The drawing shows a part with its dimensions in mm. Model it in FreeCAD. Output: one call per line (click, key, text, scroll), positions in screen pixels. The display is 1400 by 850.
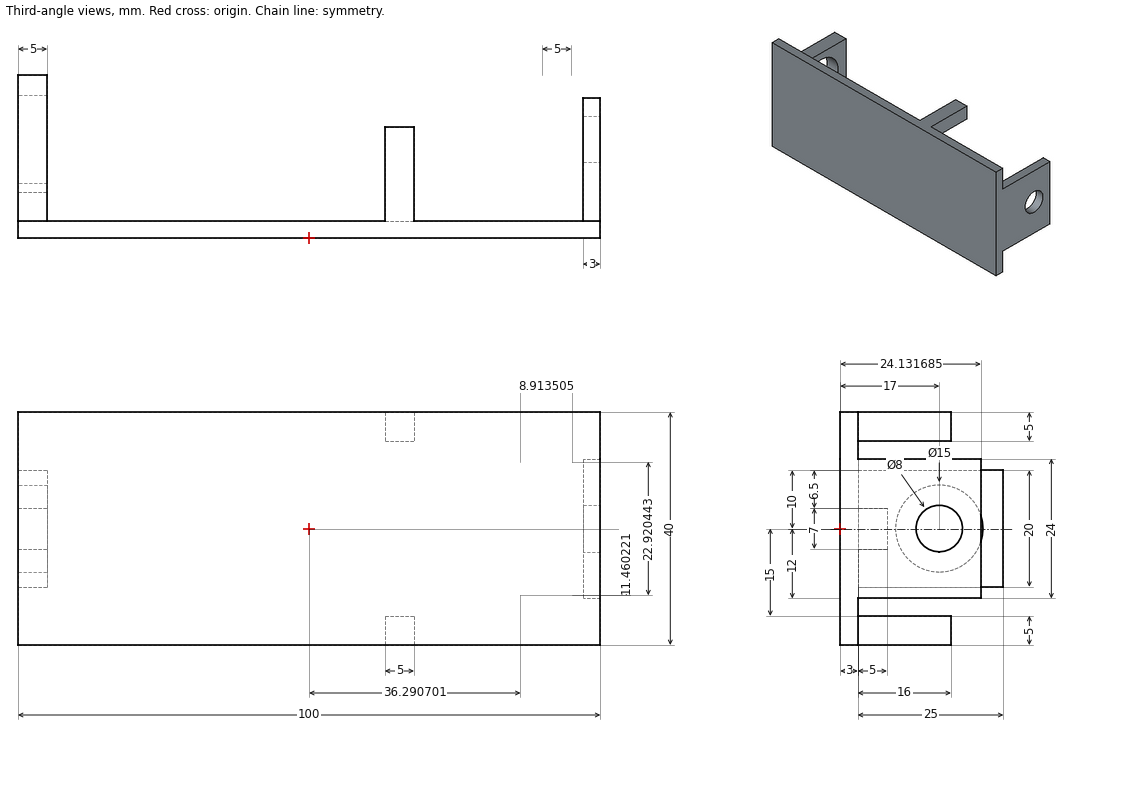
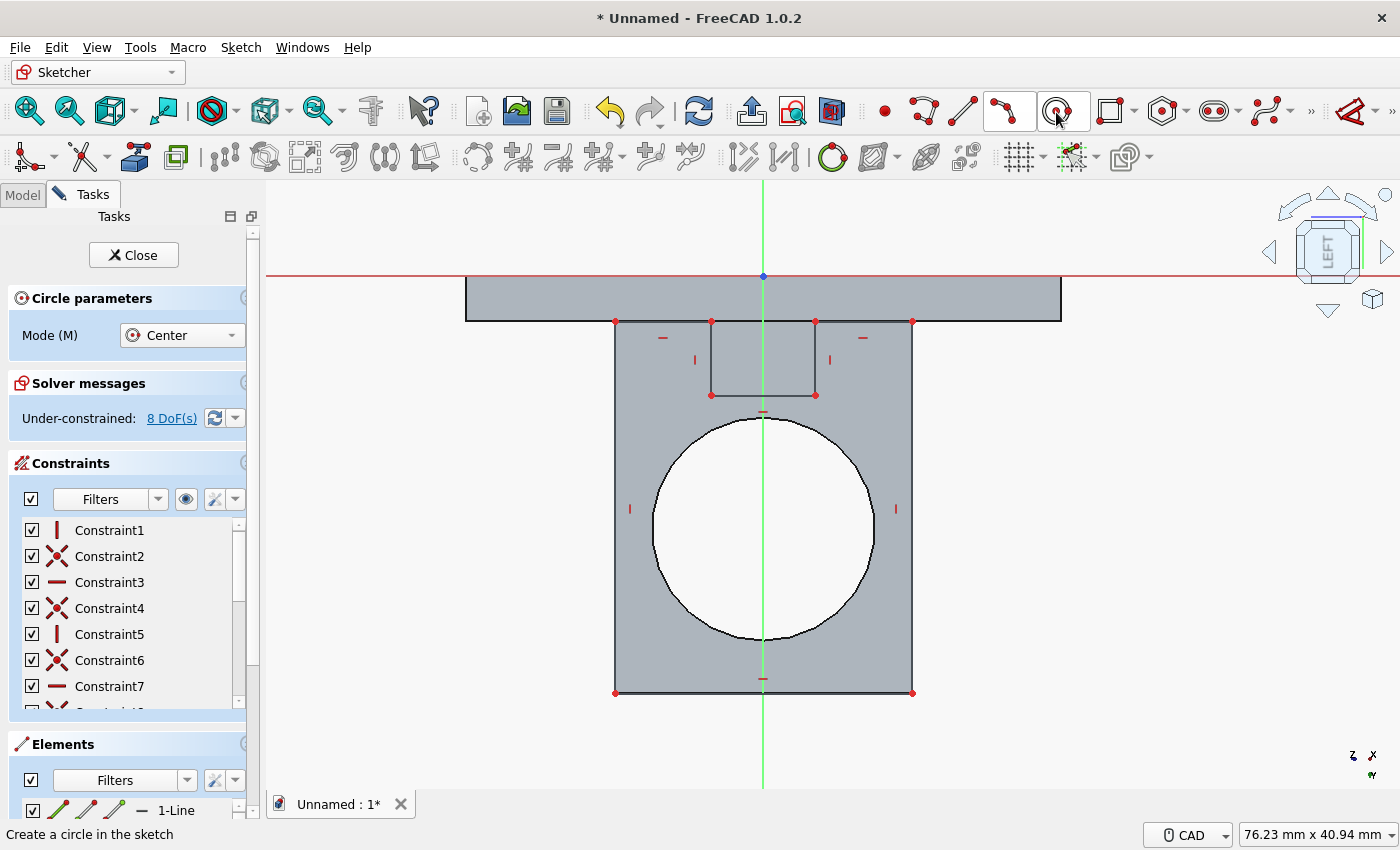
click(763, 529)
move(842, 450)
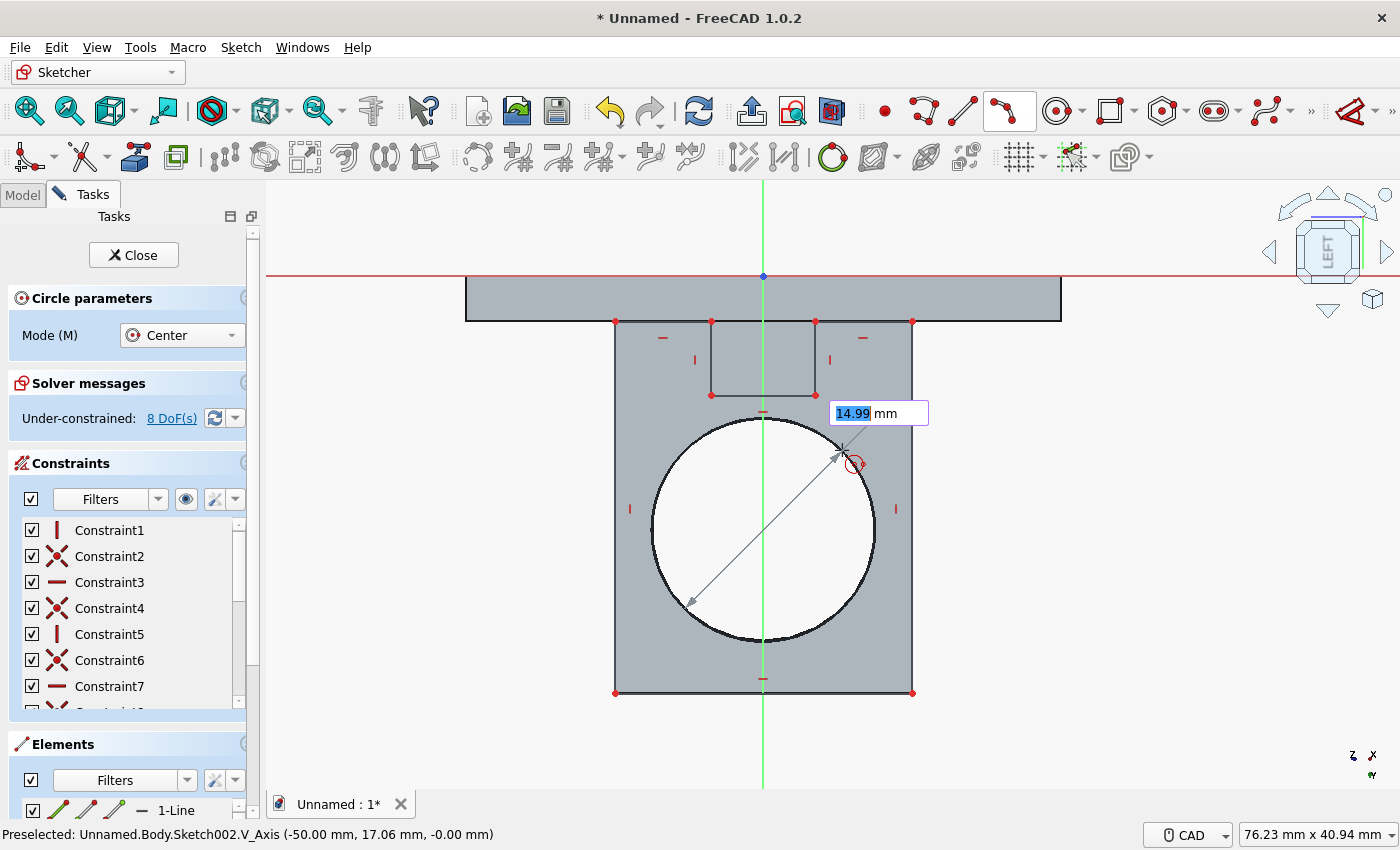
text(15)
key(Return)
key(Escape)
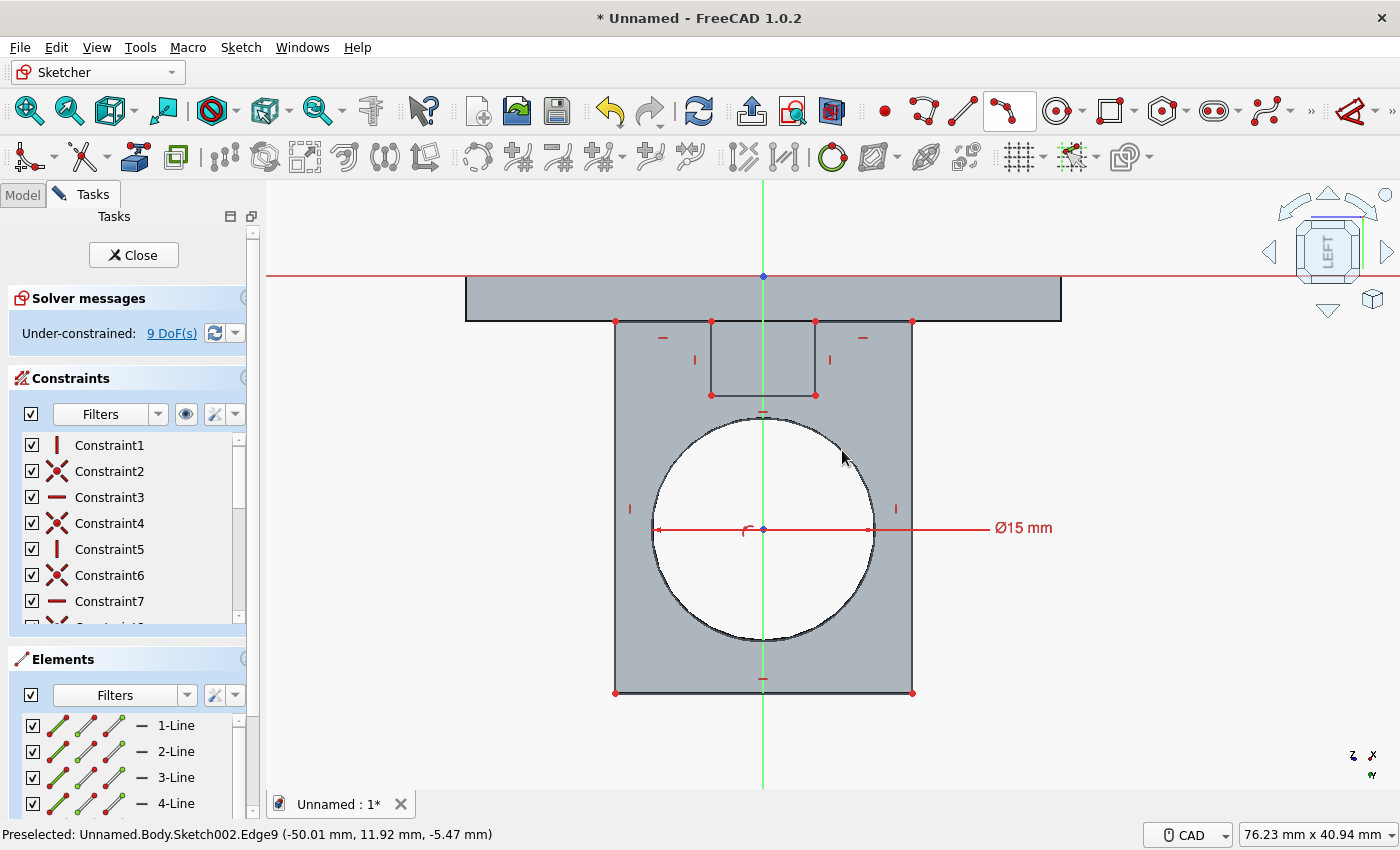
click(815, 322)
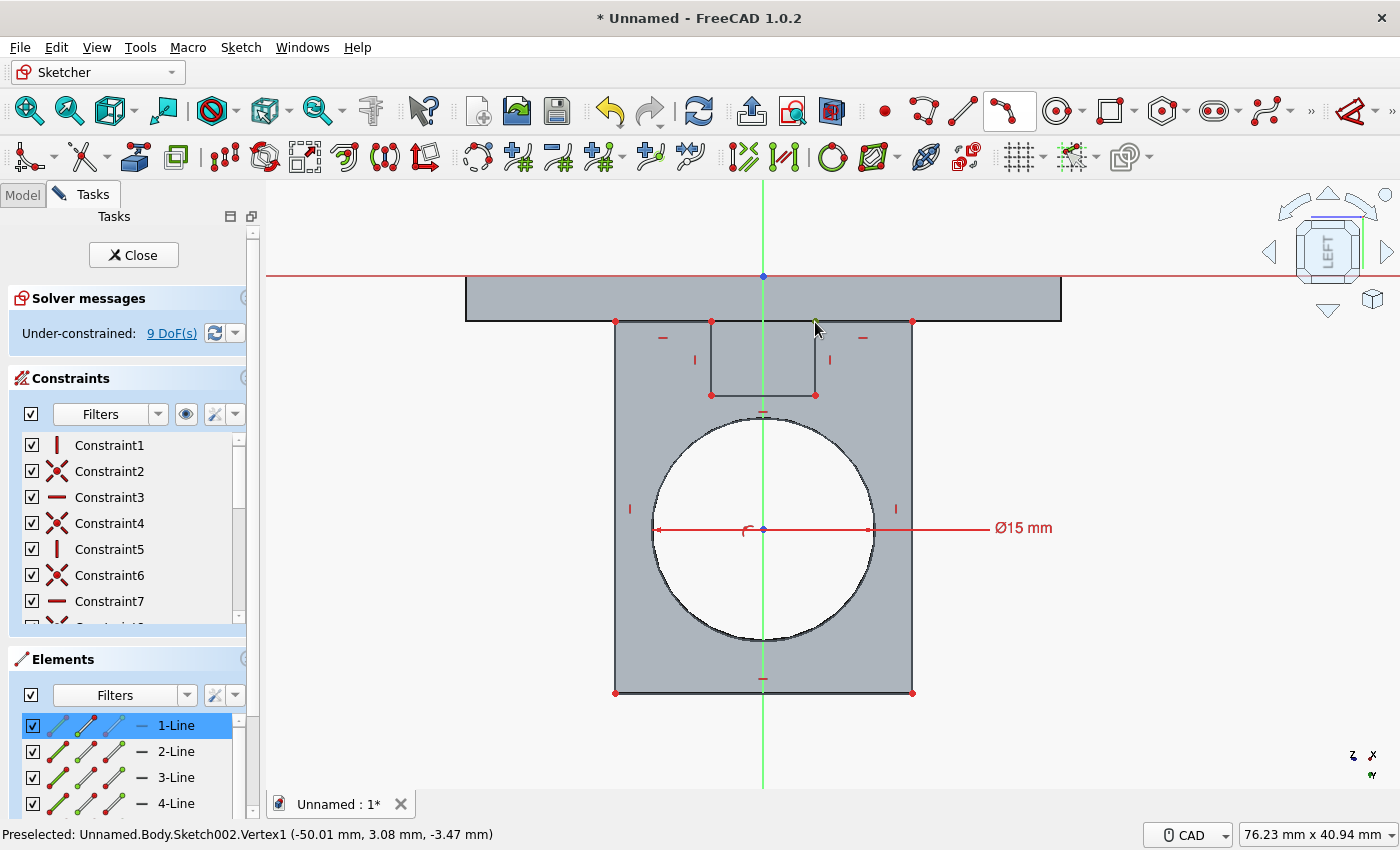
click(711, 322)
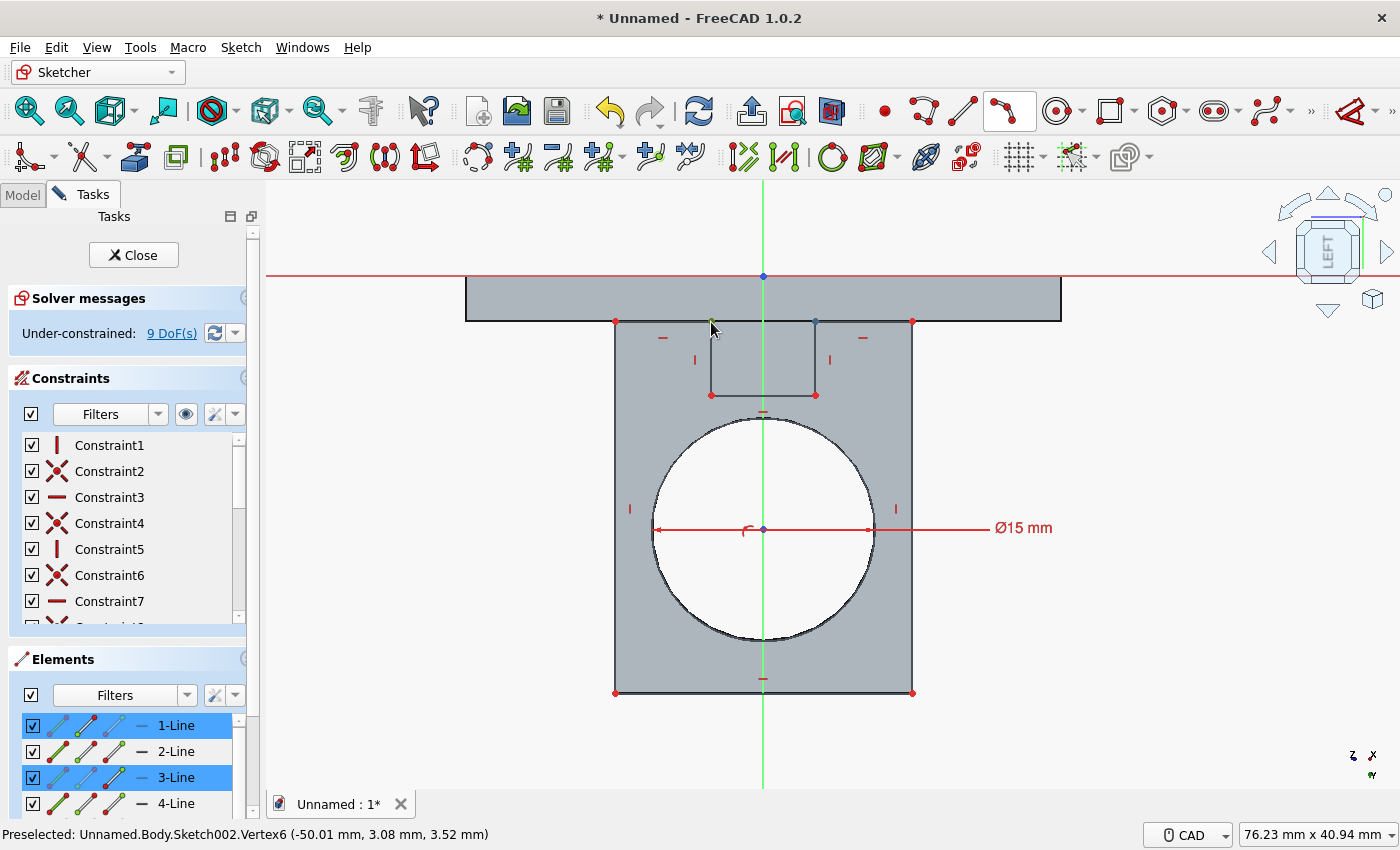
click(763, 603)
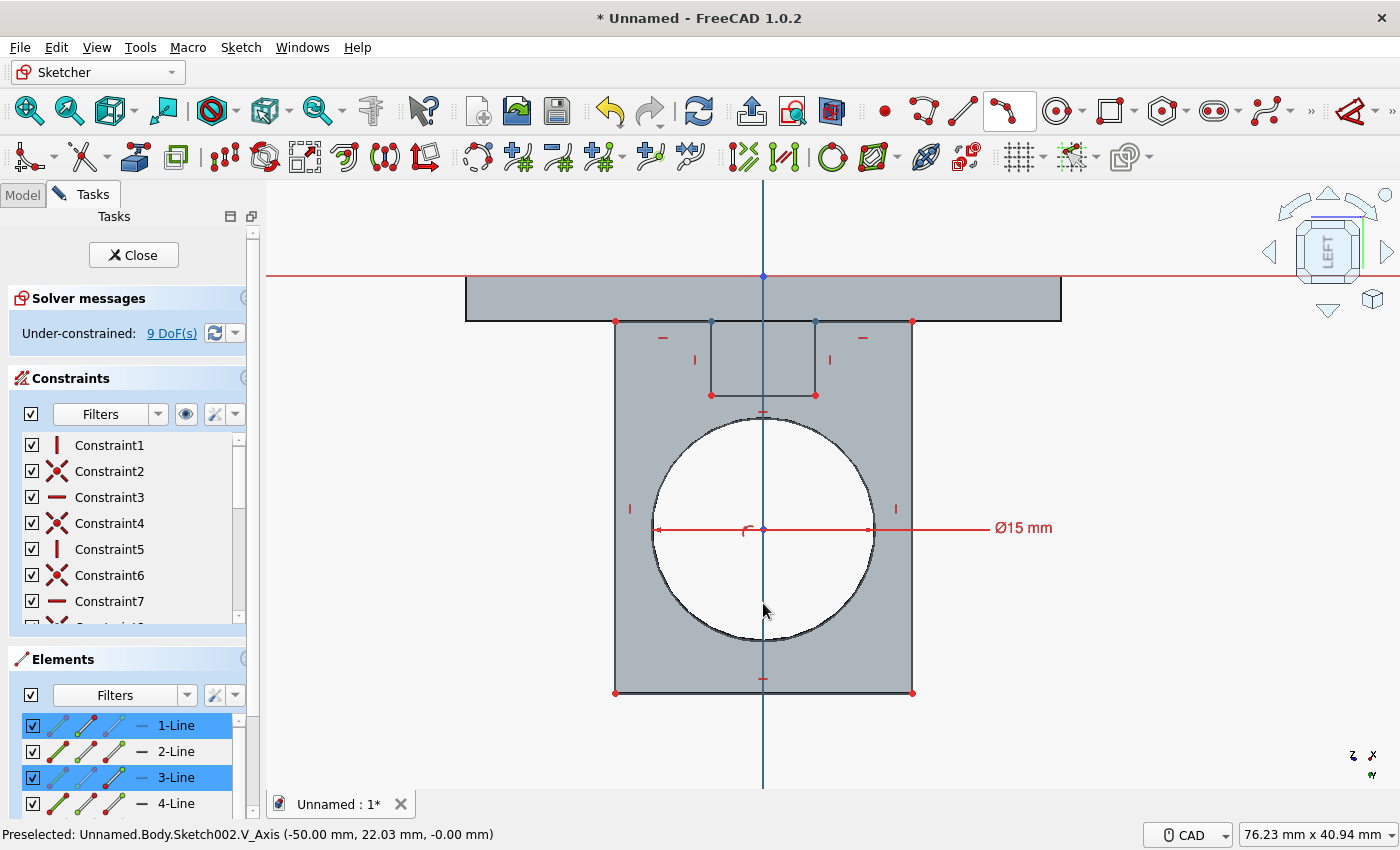
key(s)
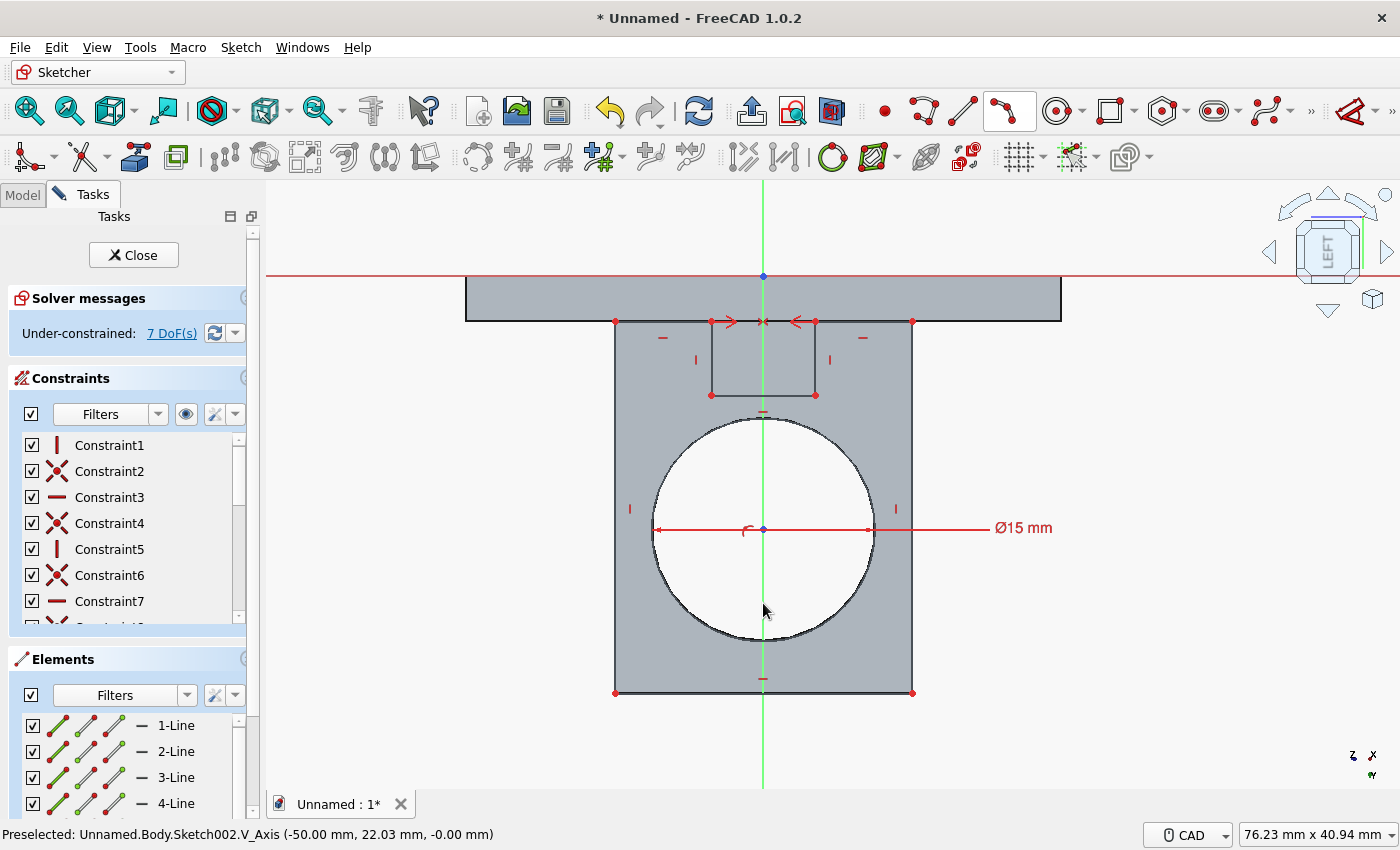
click(1350, 112)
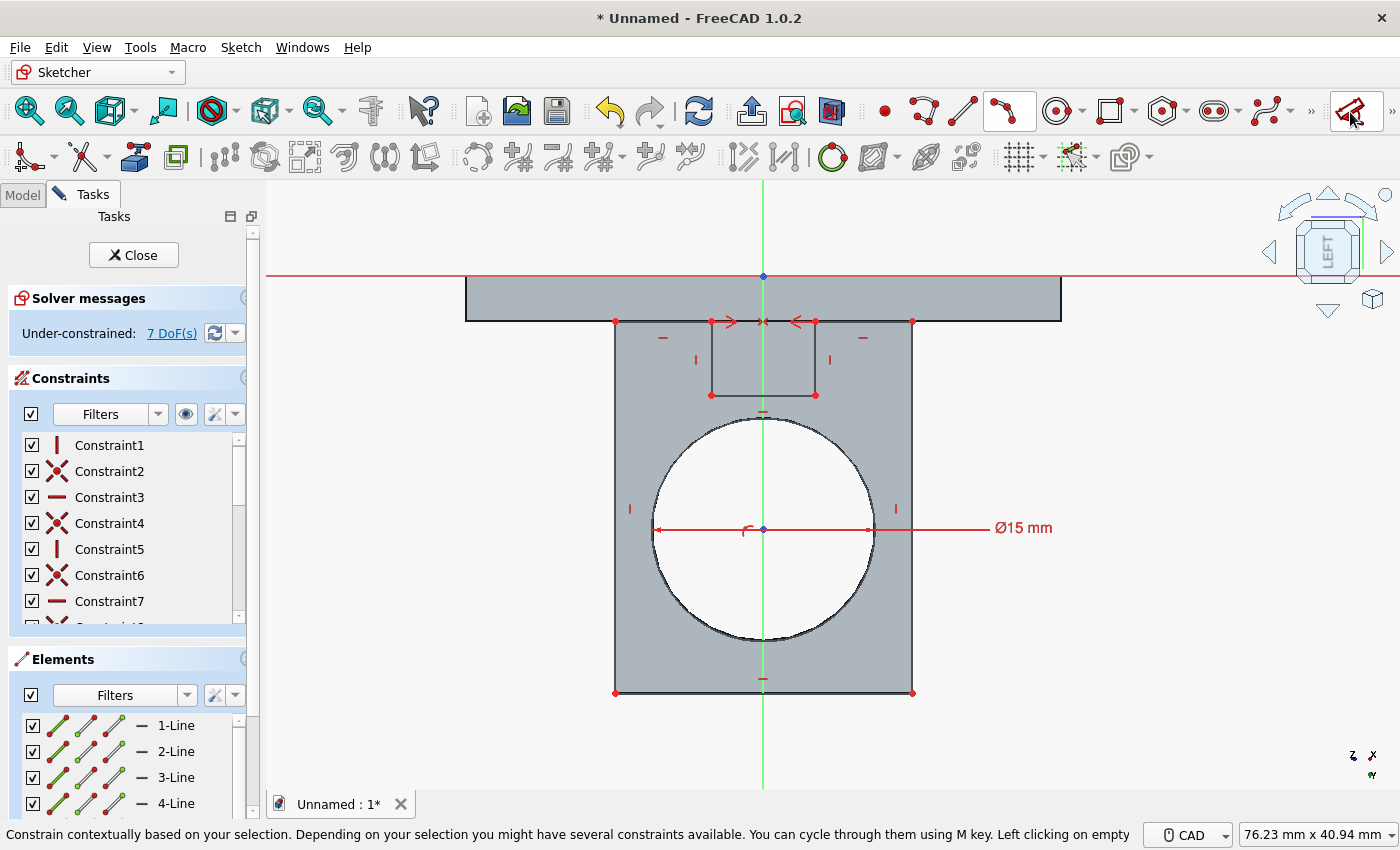
click(815, 344)
click(849, 359)